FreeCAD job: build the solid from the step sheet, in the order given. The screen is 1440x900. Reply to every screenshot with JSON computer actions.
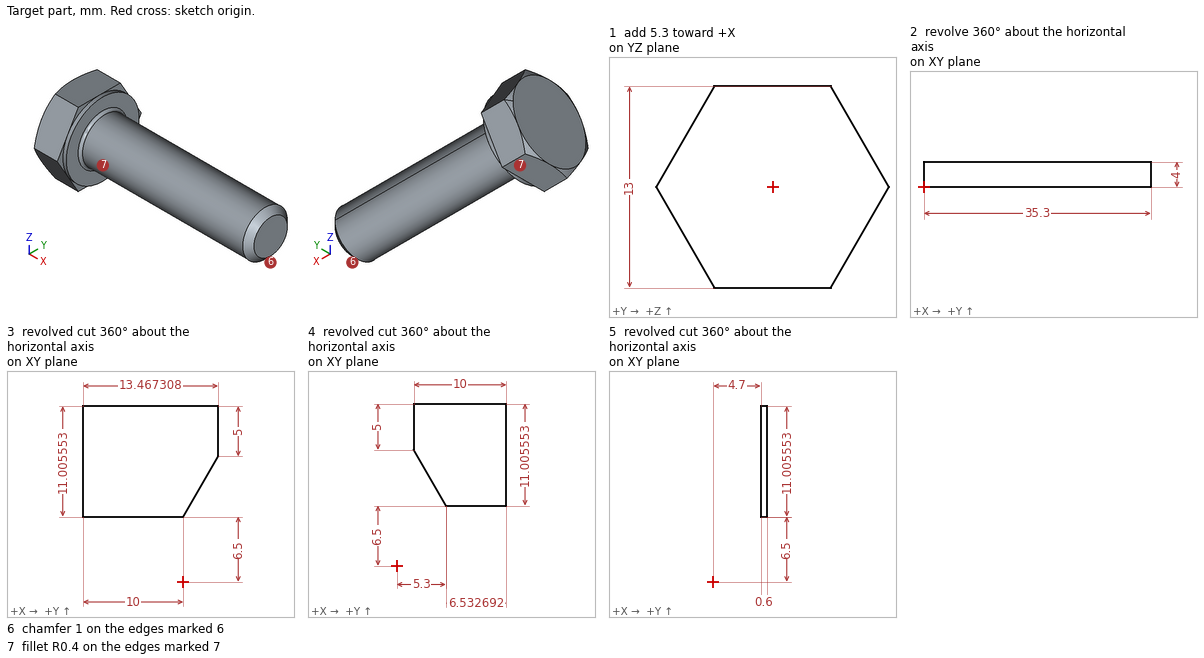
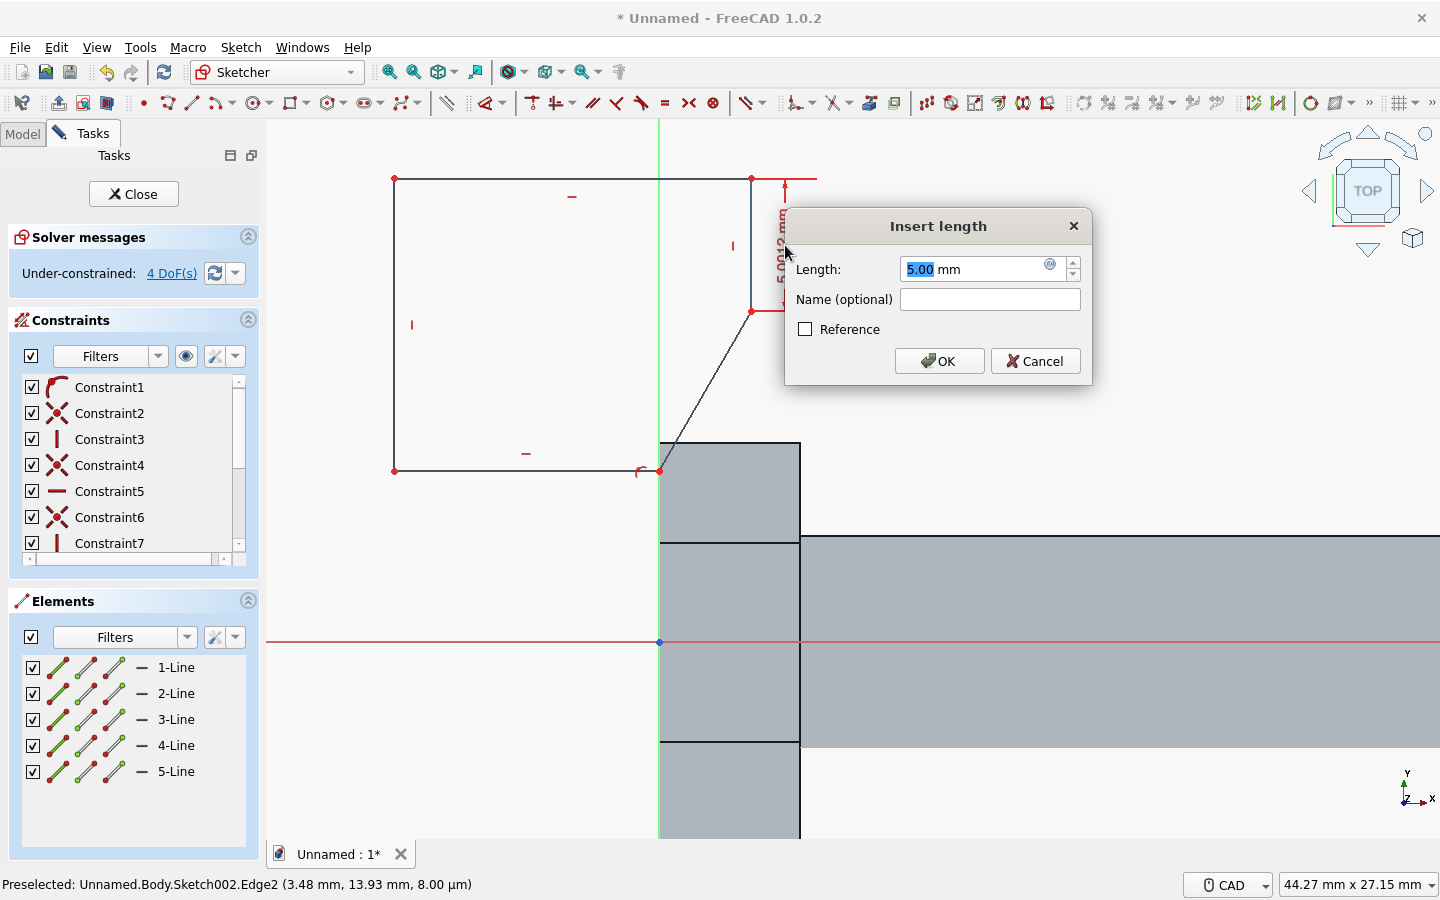
{"action": "type", "text": "5"}
{"action": "key", "text": "Return"}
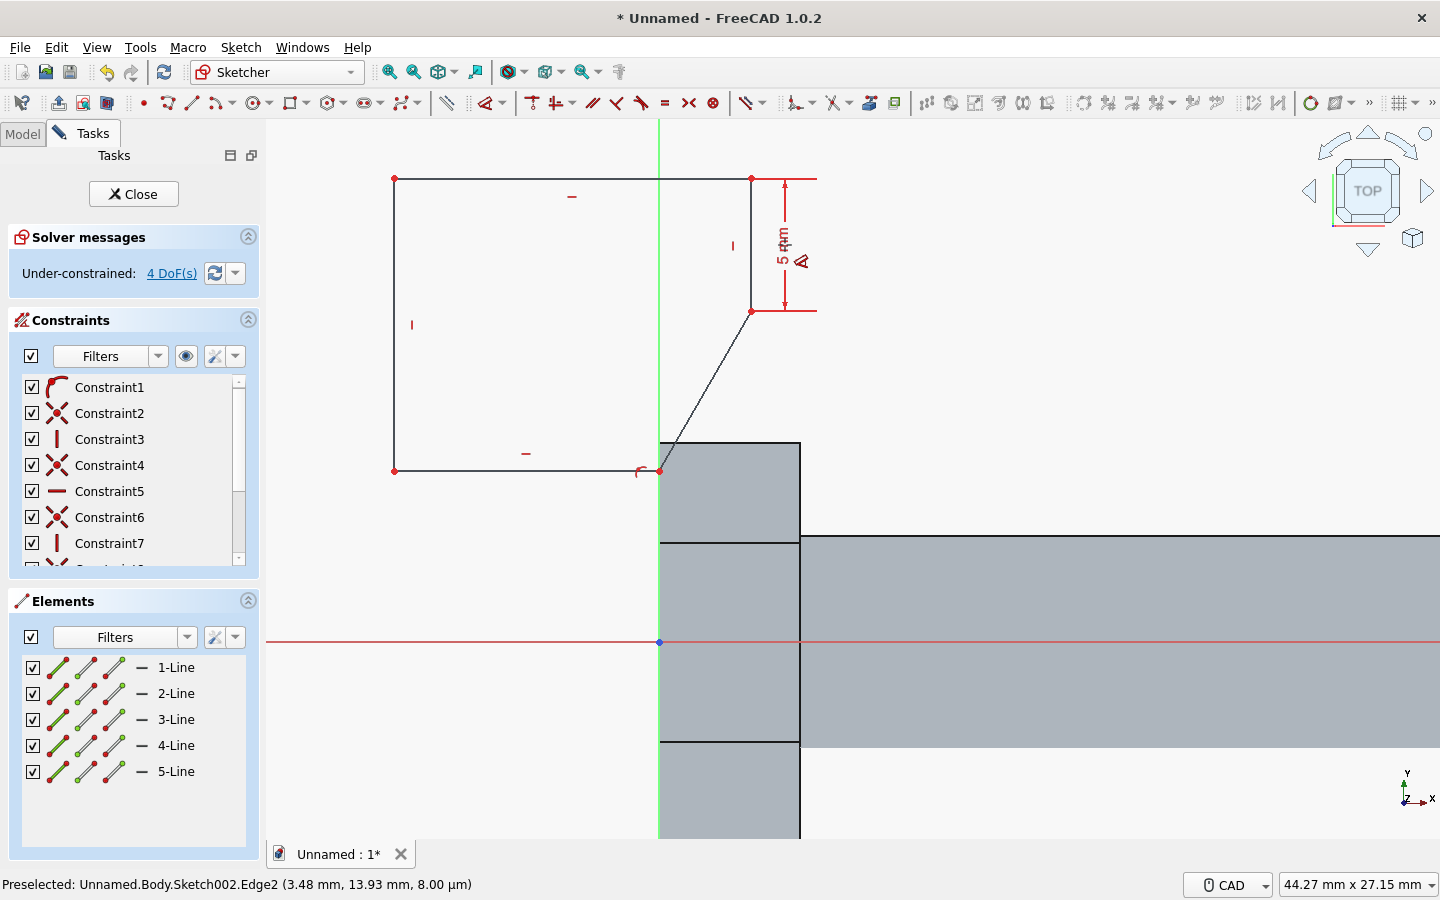
{"action": "left_click", "coordinate": [474, 471]}
{"action": "left_click", "coordinate": [527, 505]}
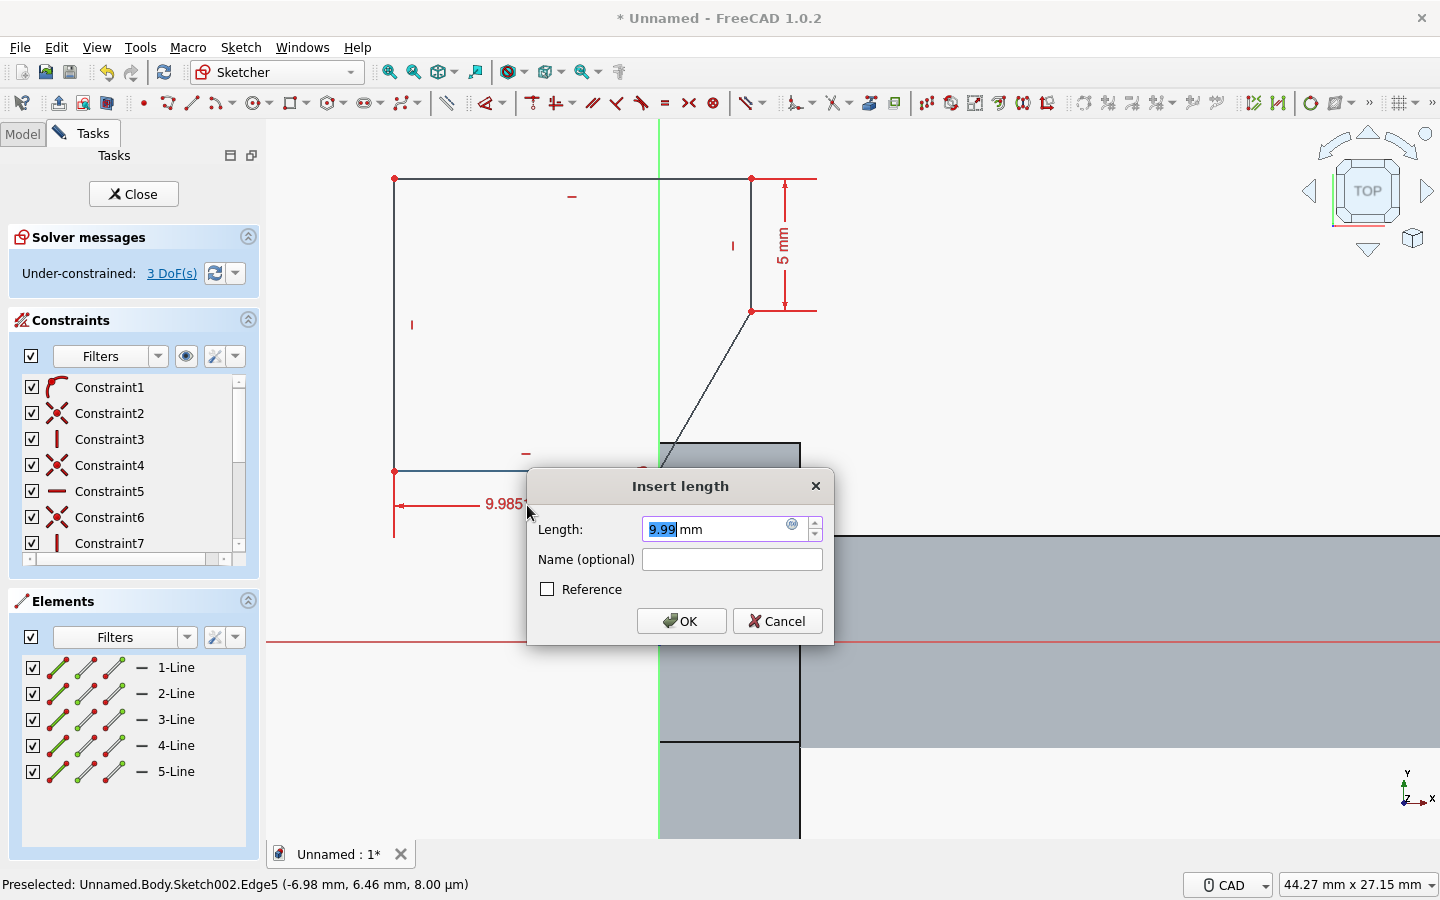
{"action": "type", "text": "10"}
{"action": "key", "text": "Return"}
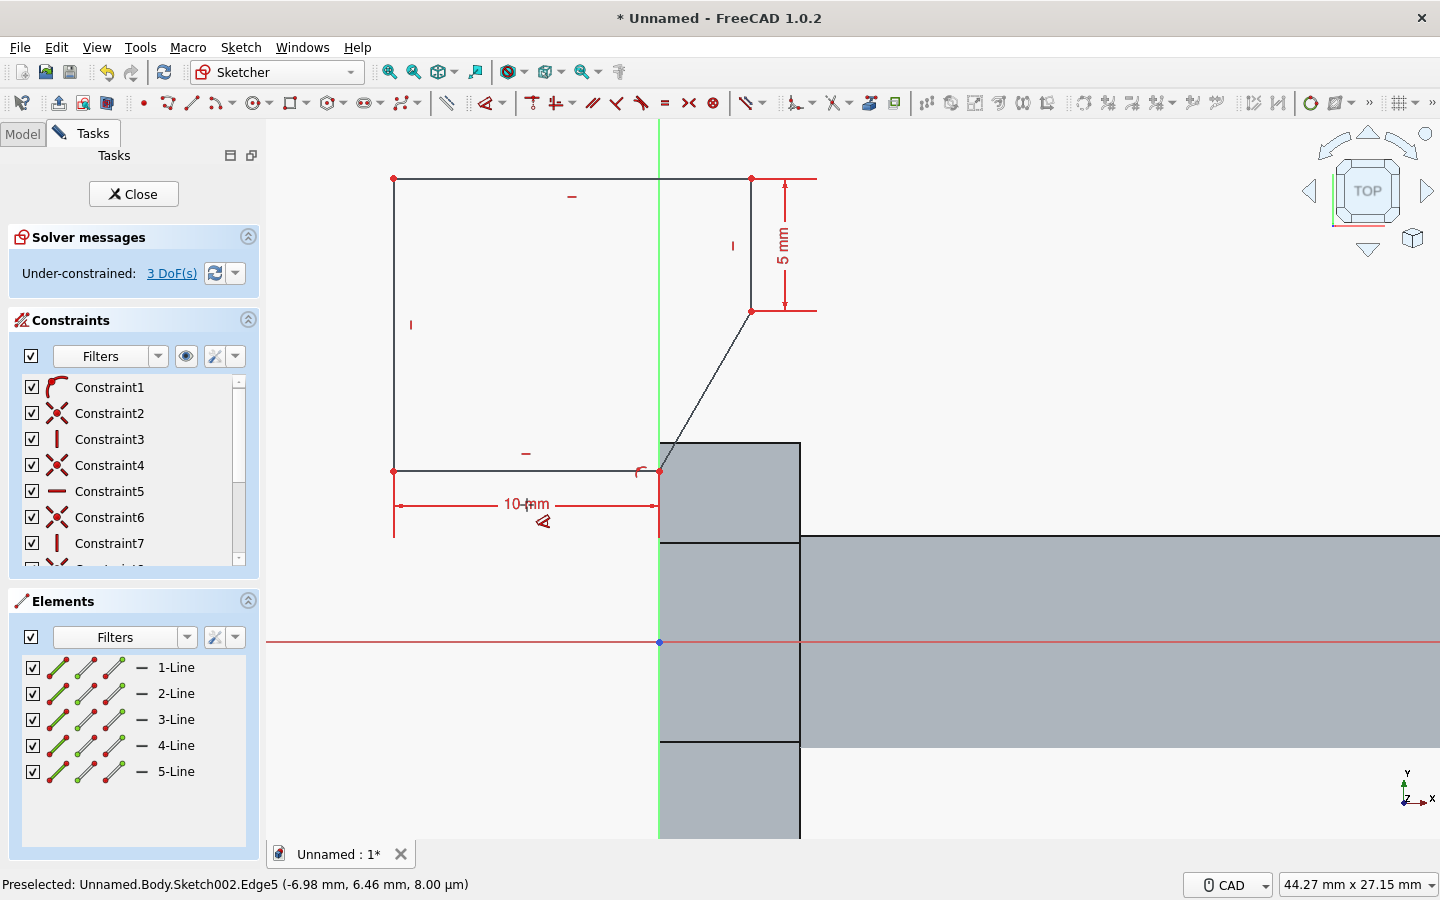
{"action": "left_click", "coordinate": [659, 471]}
{"action": "left_click", "coordinate": [693, 557]}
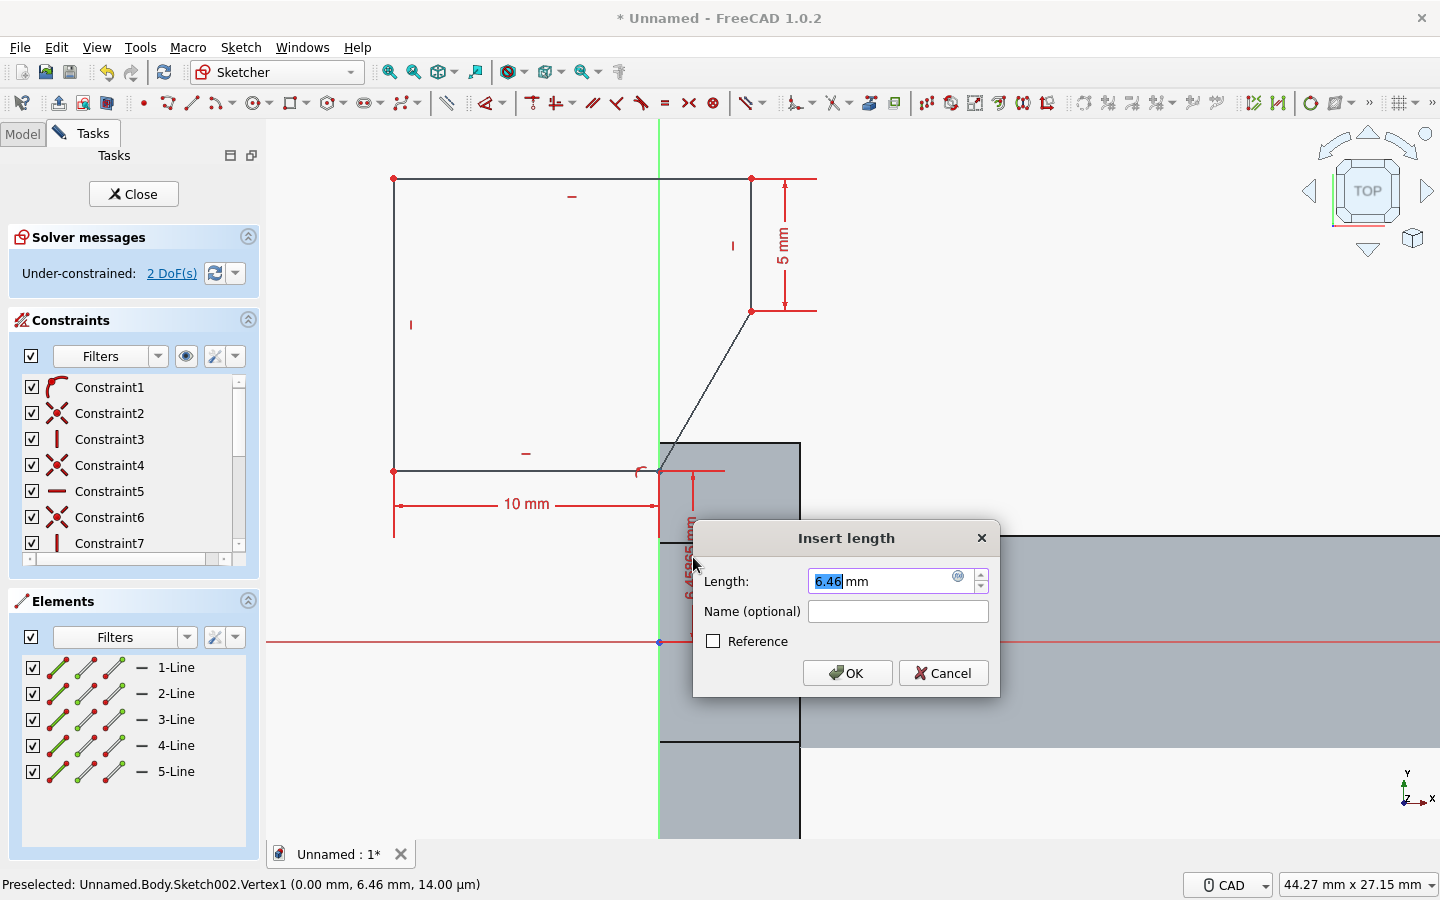
{"action": "type", "text": "6.5"}
{"action": "key", "text": "Return"}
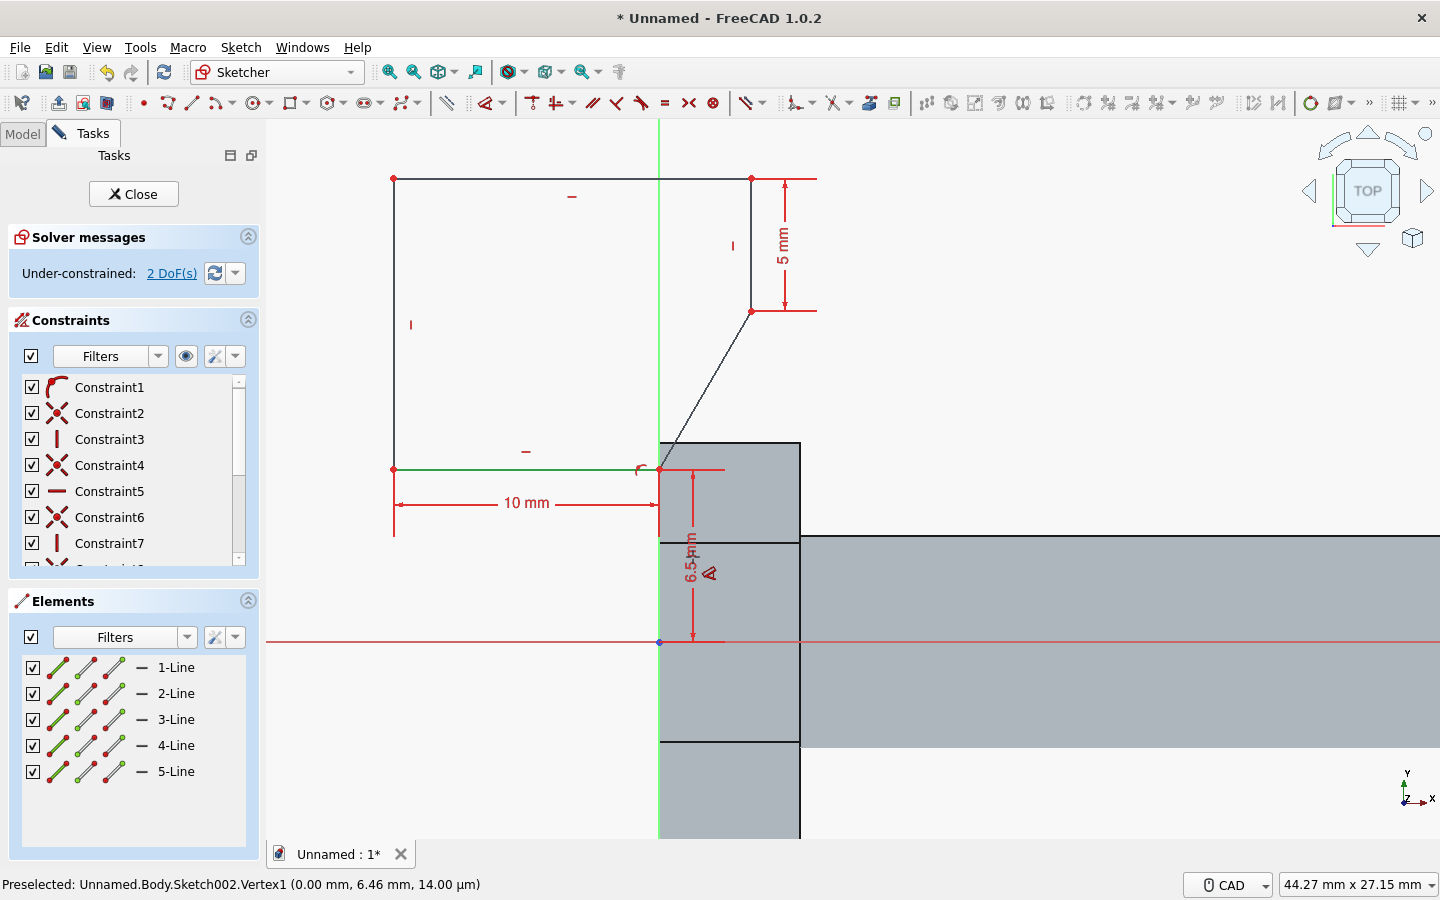
{"action": "left_click", "coordinate": [644, 179]}
{"action": "left_click", "coordinate": [573, 213]}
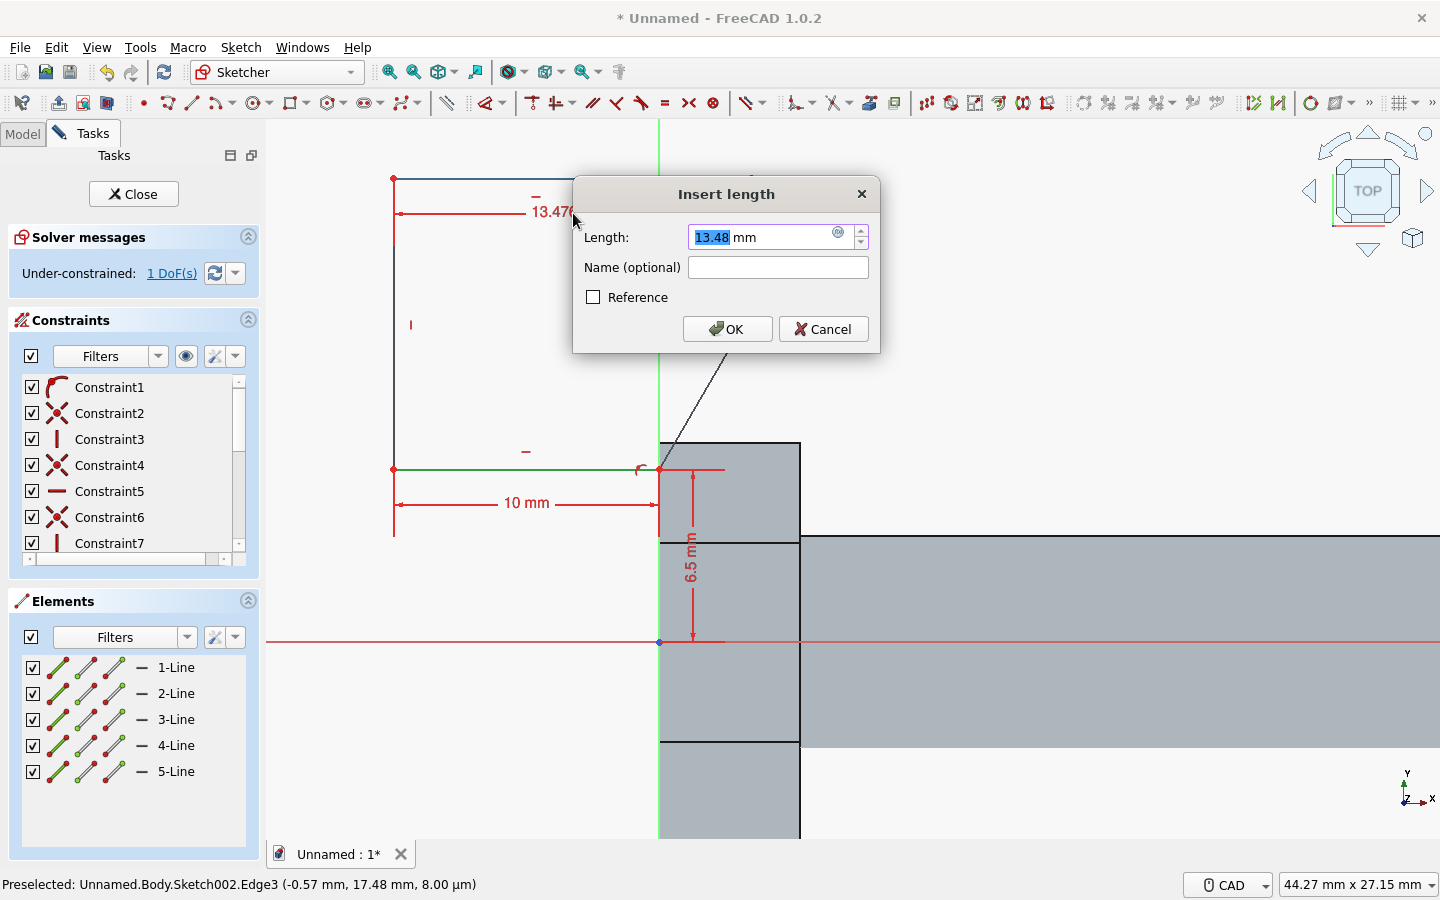
{"action": "type", "text": "13.467308"}
{"action": "key", "text": "Return"}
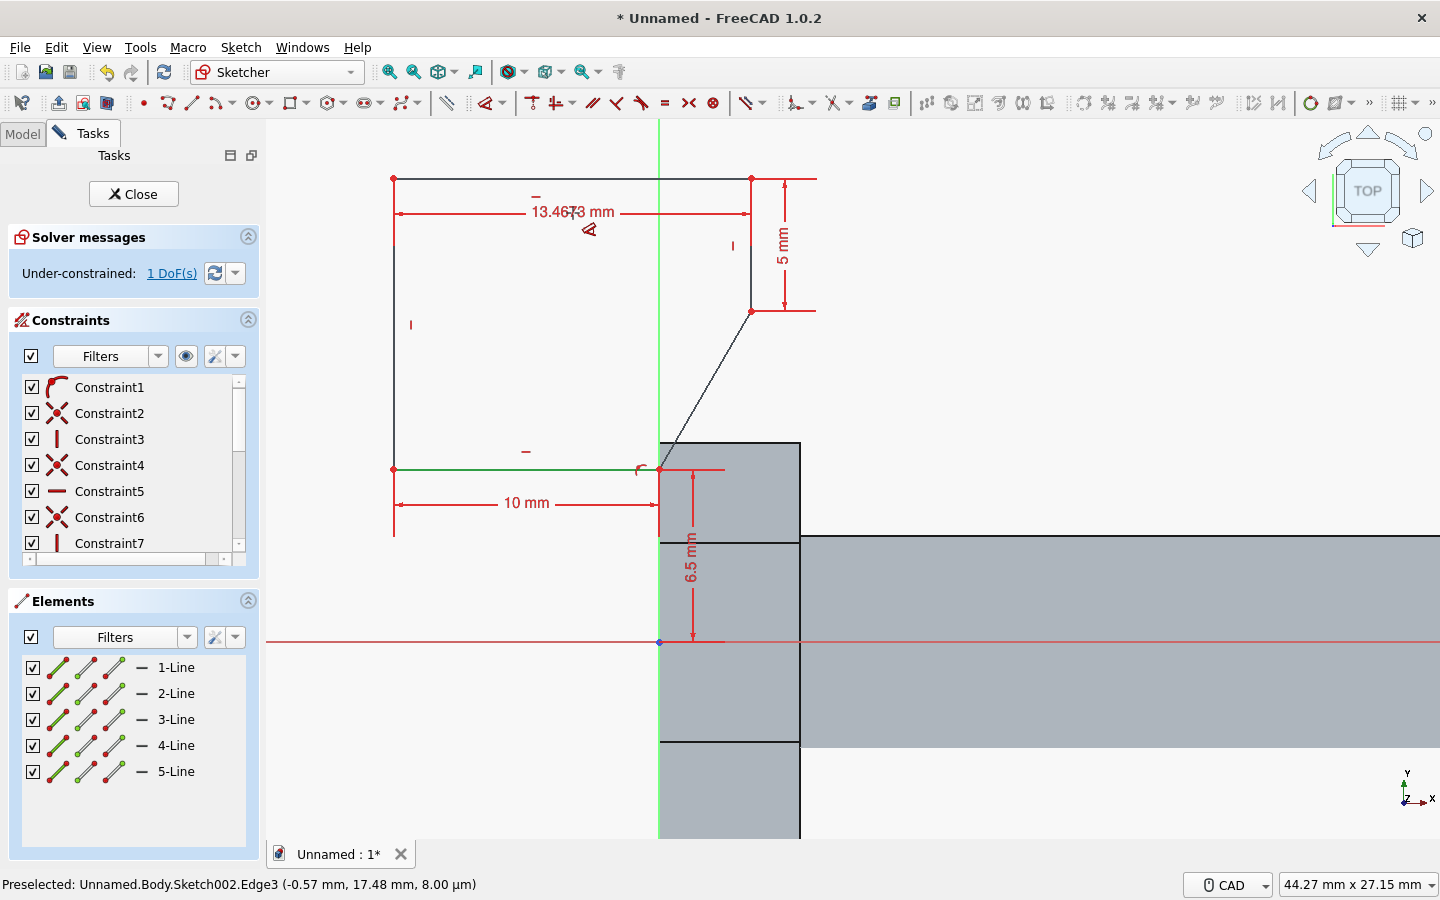
{"action": "left_click", "coordinate": [394, 266]}
{"action": "left_click", "coordinate": [360, 324]}